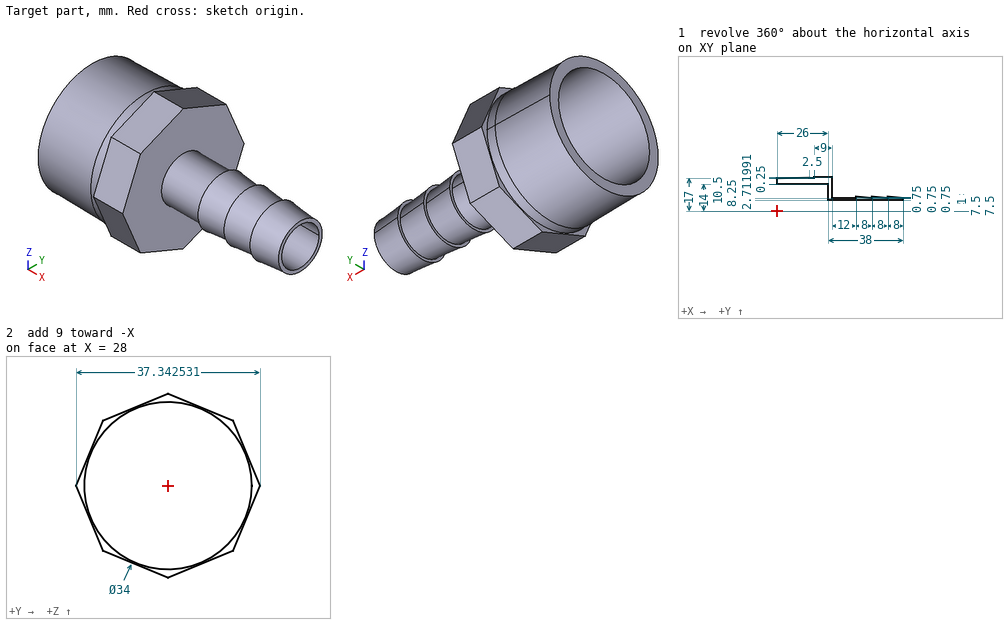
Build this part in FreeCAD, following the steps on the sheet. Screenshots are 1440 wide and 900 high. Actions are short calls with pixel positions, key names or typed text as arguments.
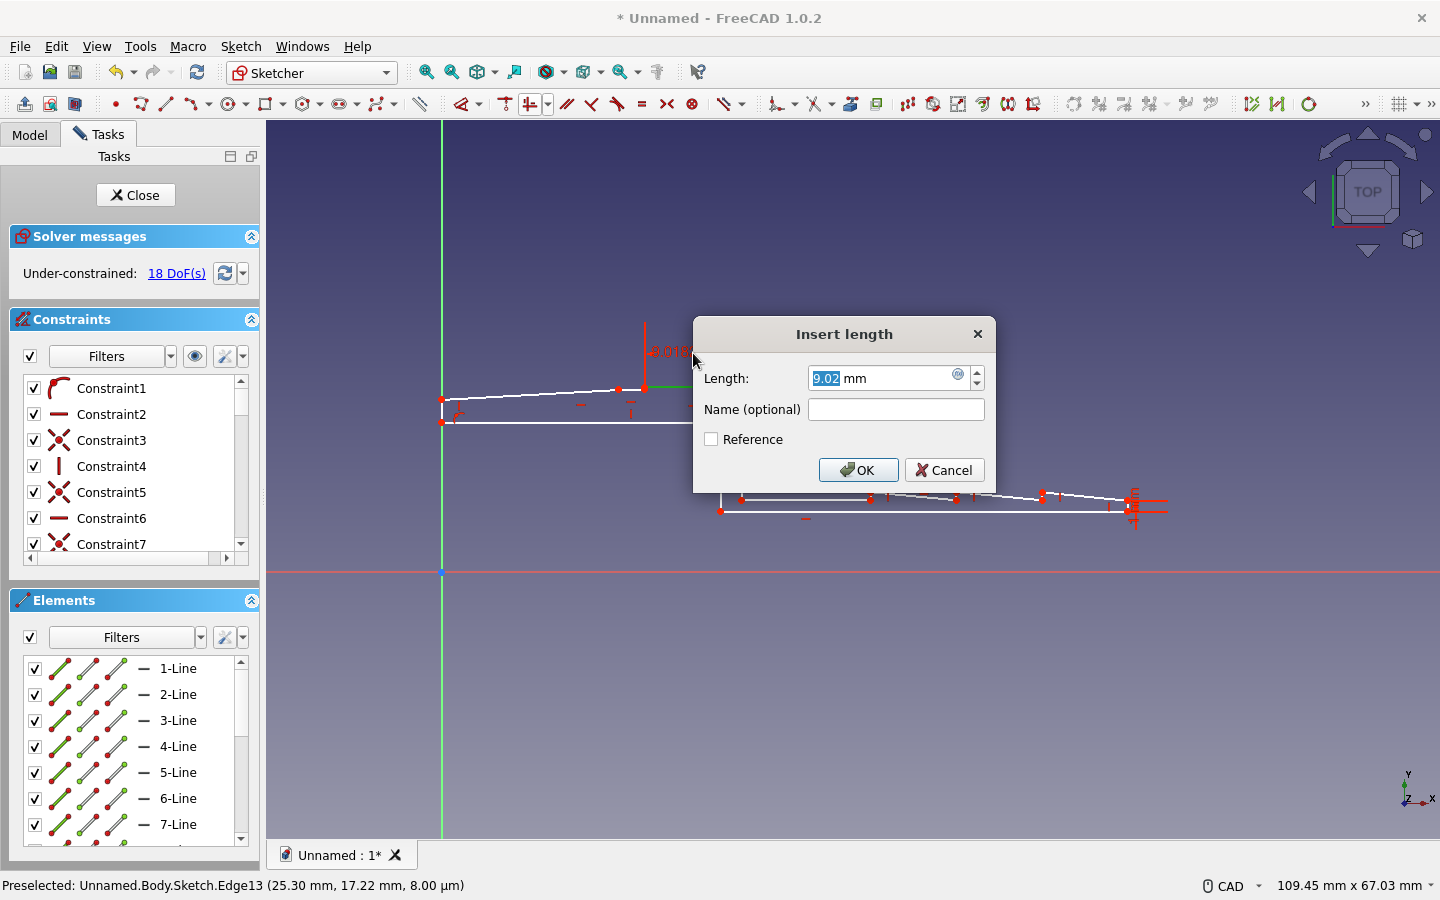
text(9)
key(Return)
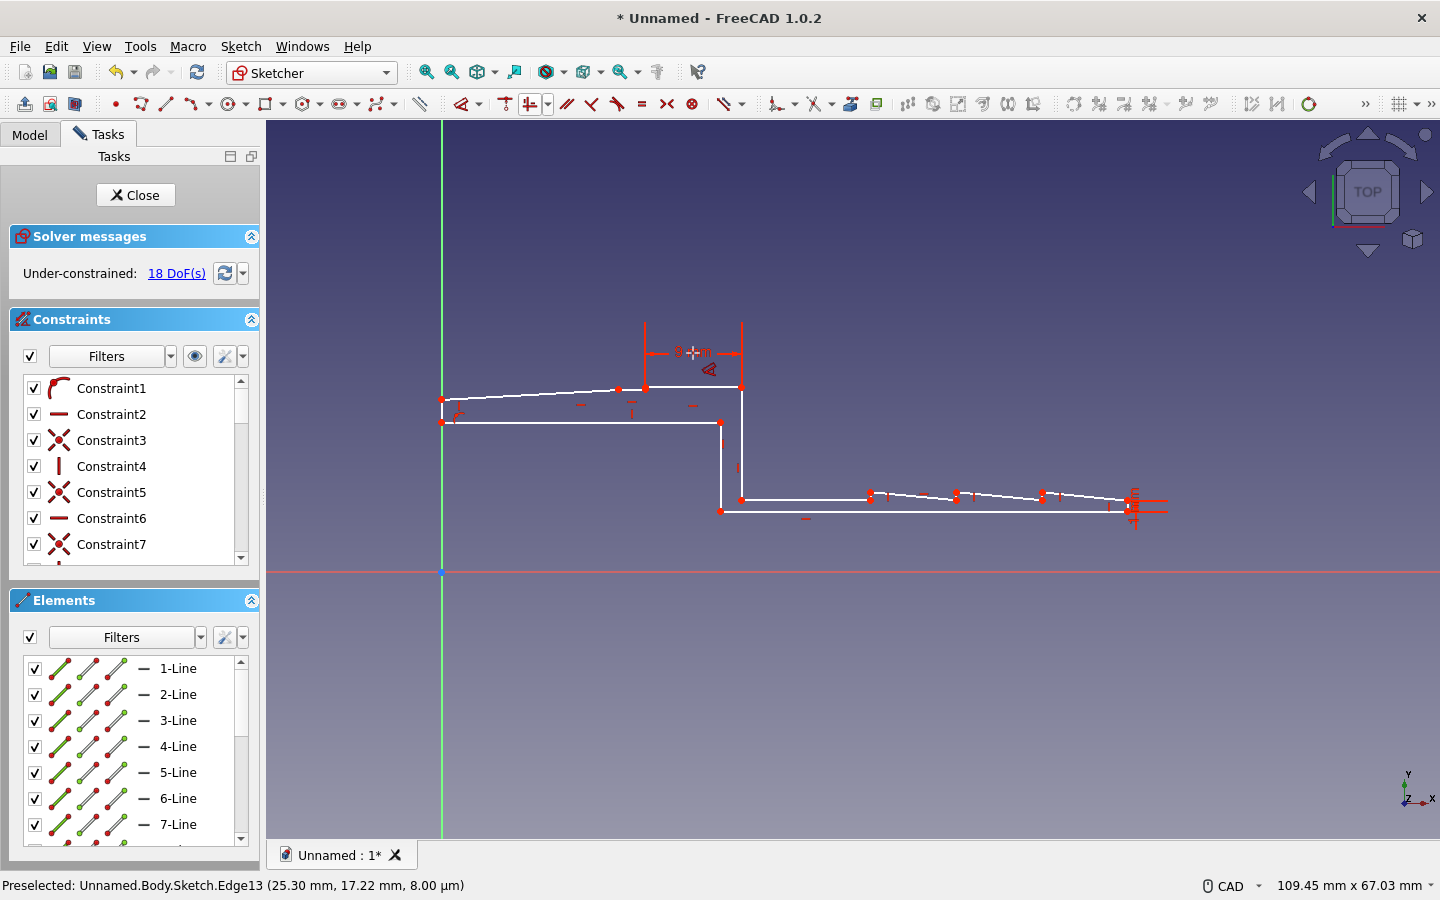
click(525, 423)
click(581, 457)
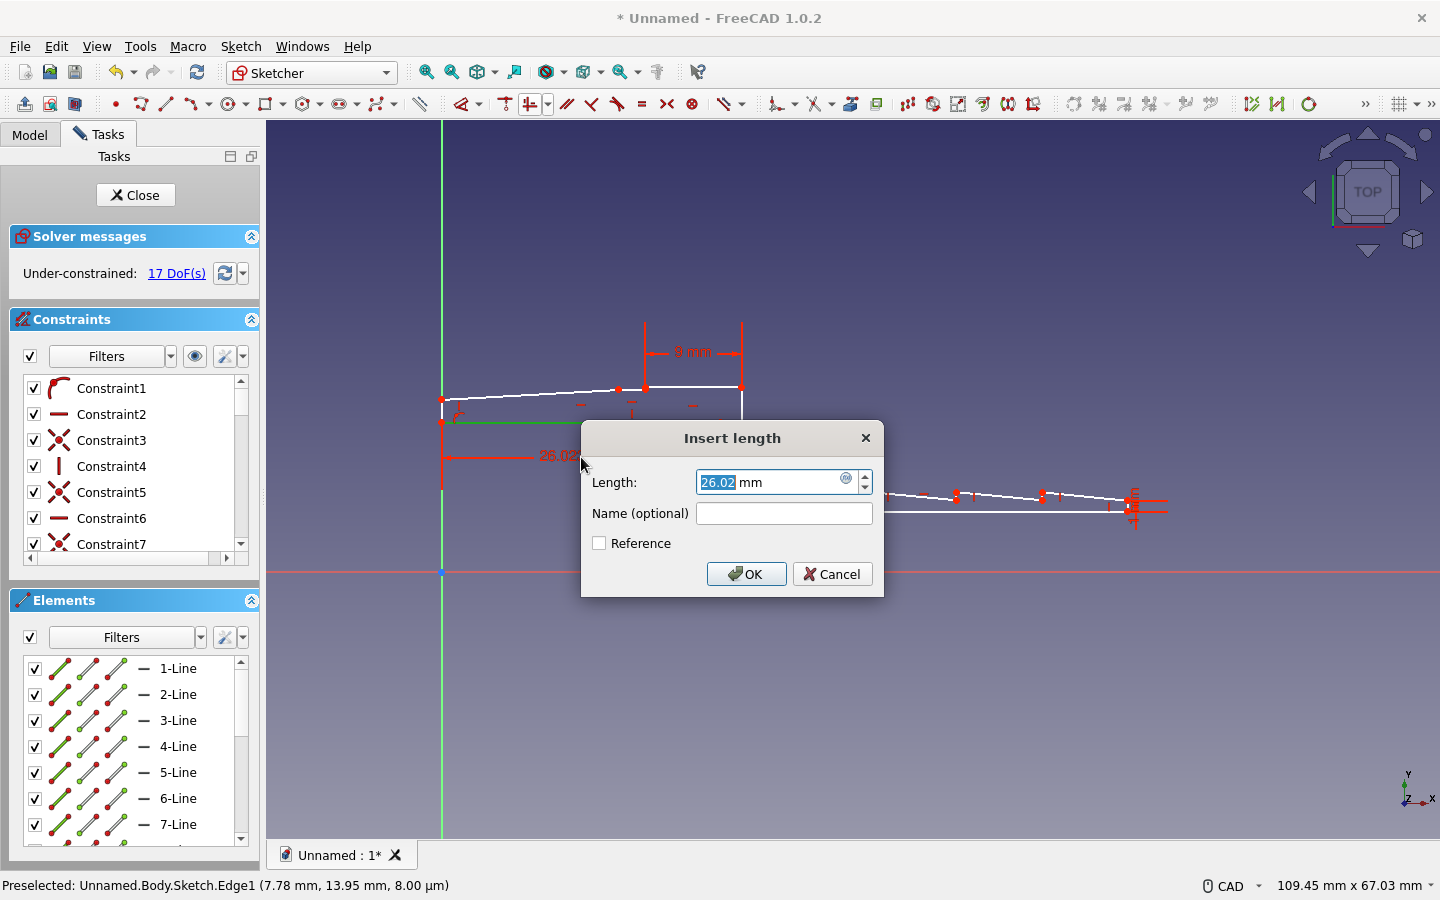
text(26)
key(Return)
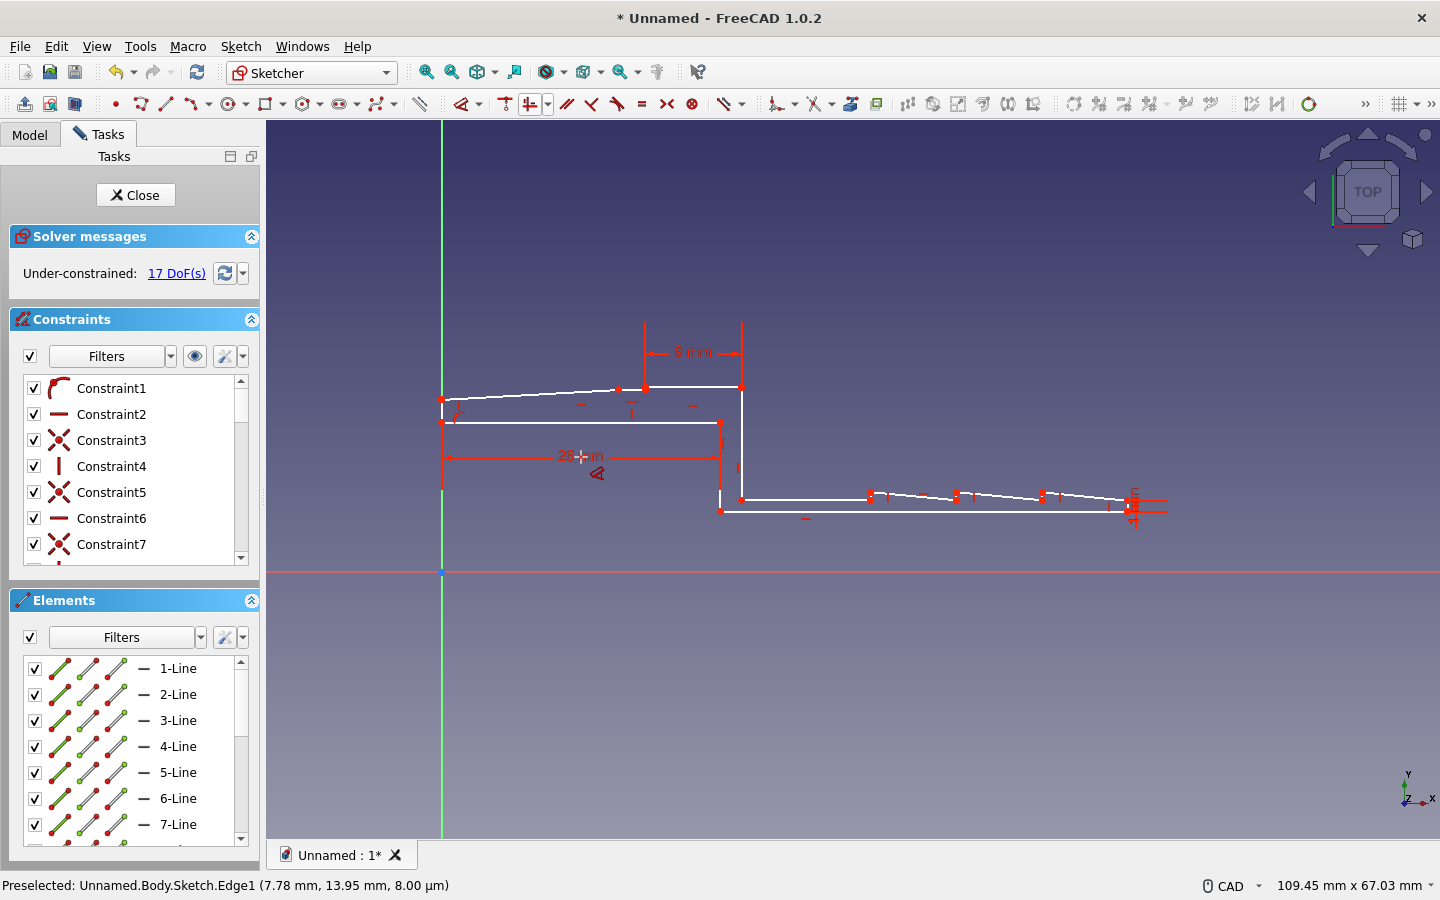
scroll(843, 512, up, 2)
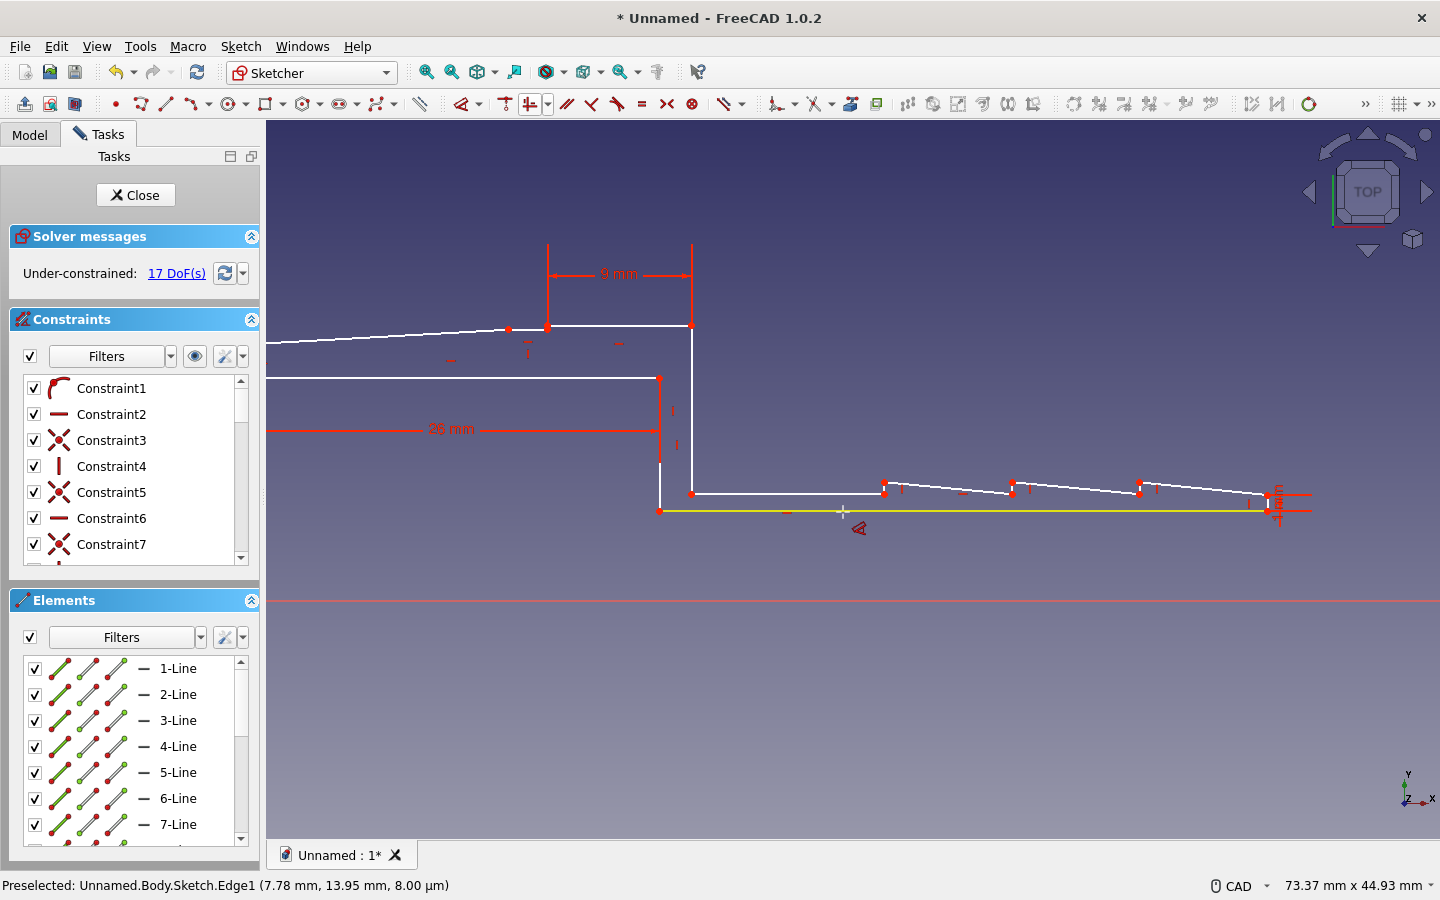
click(842, 511)
click(964, 545)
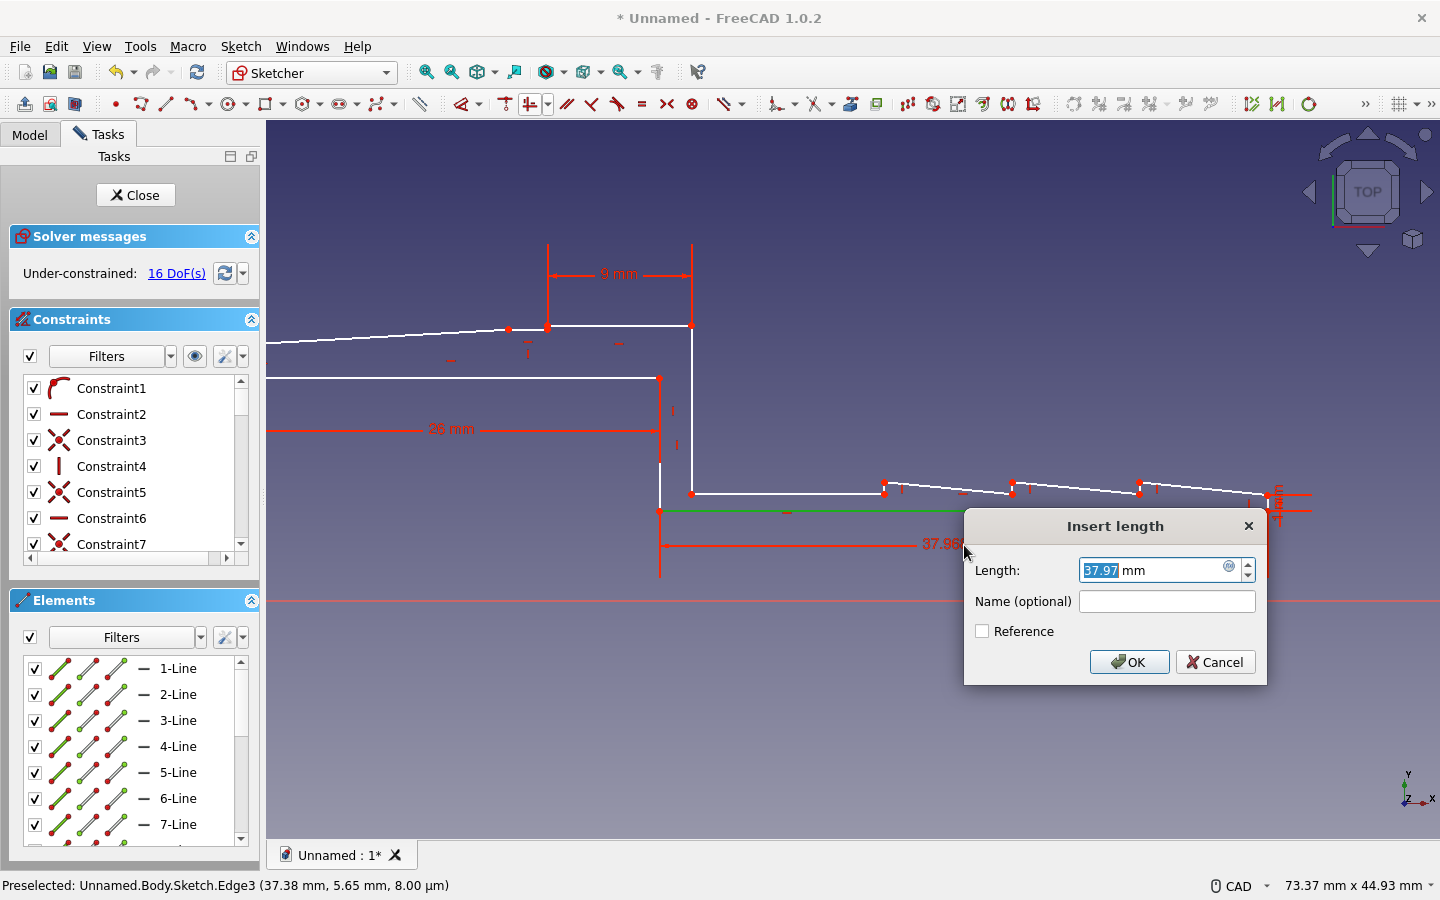
text(38)
key(Return)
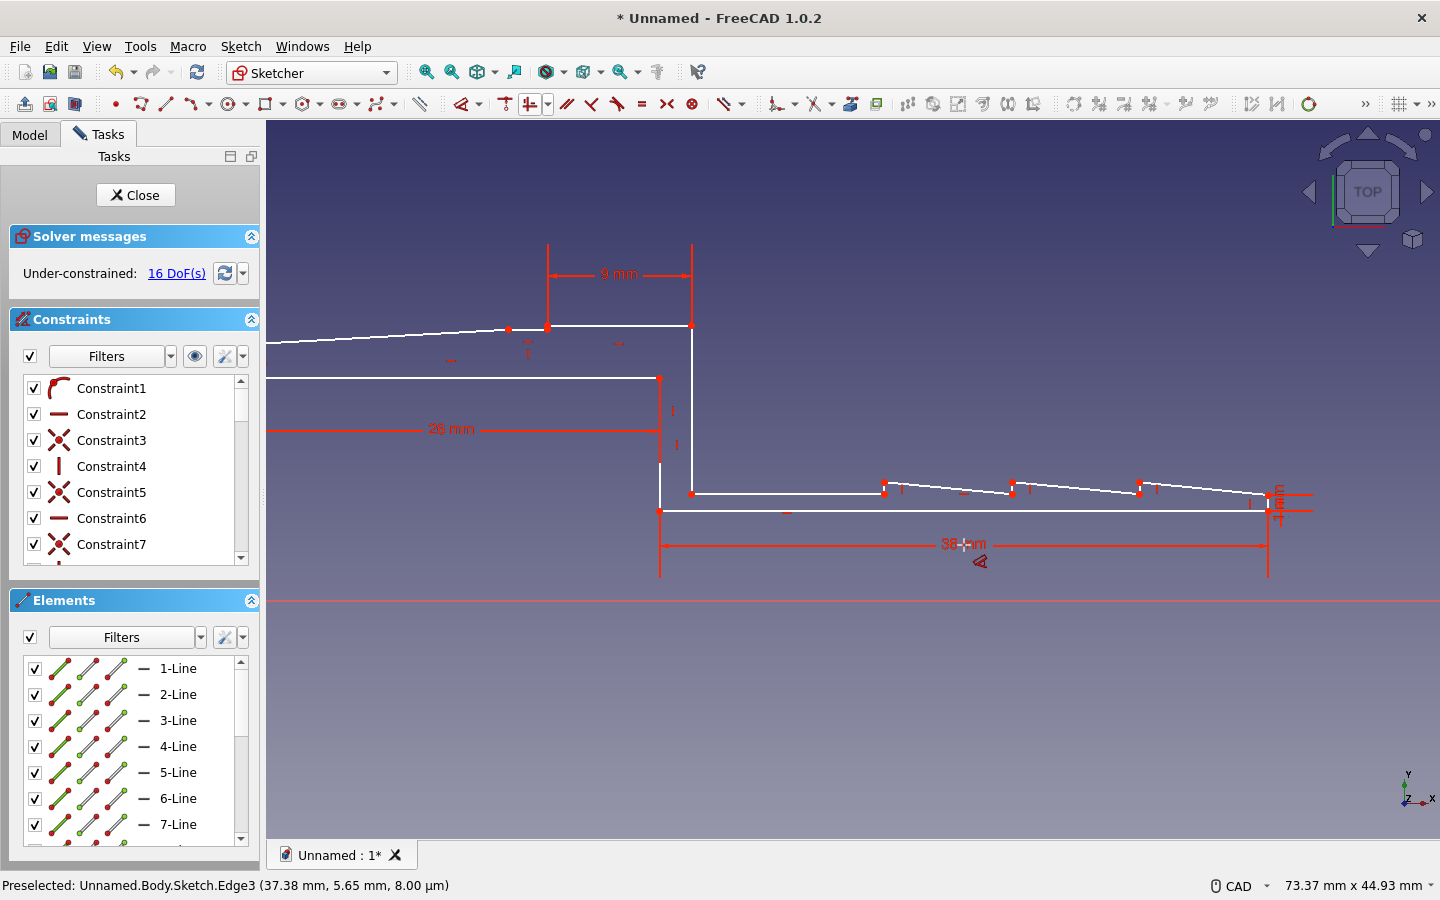
click(826, 494)
click(788, 528)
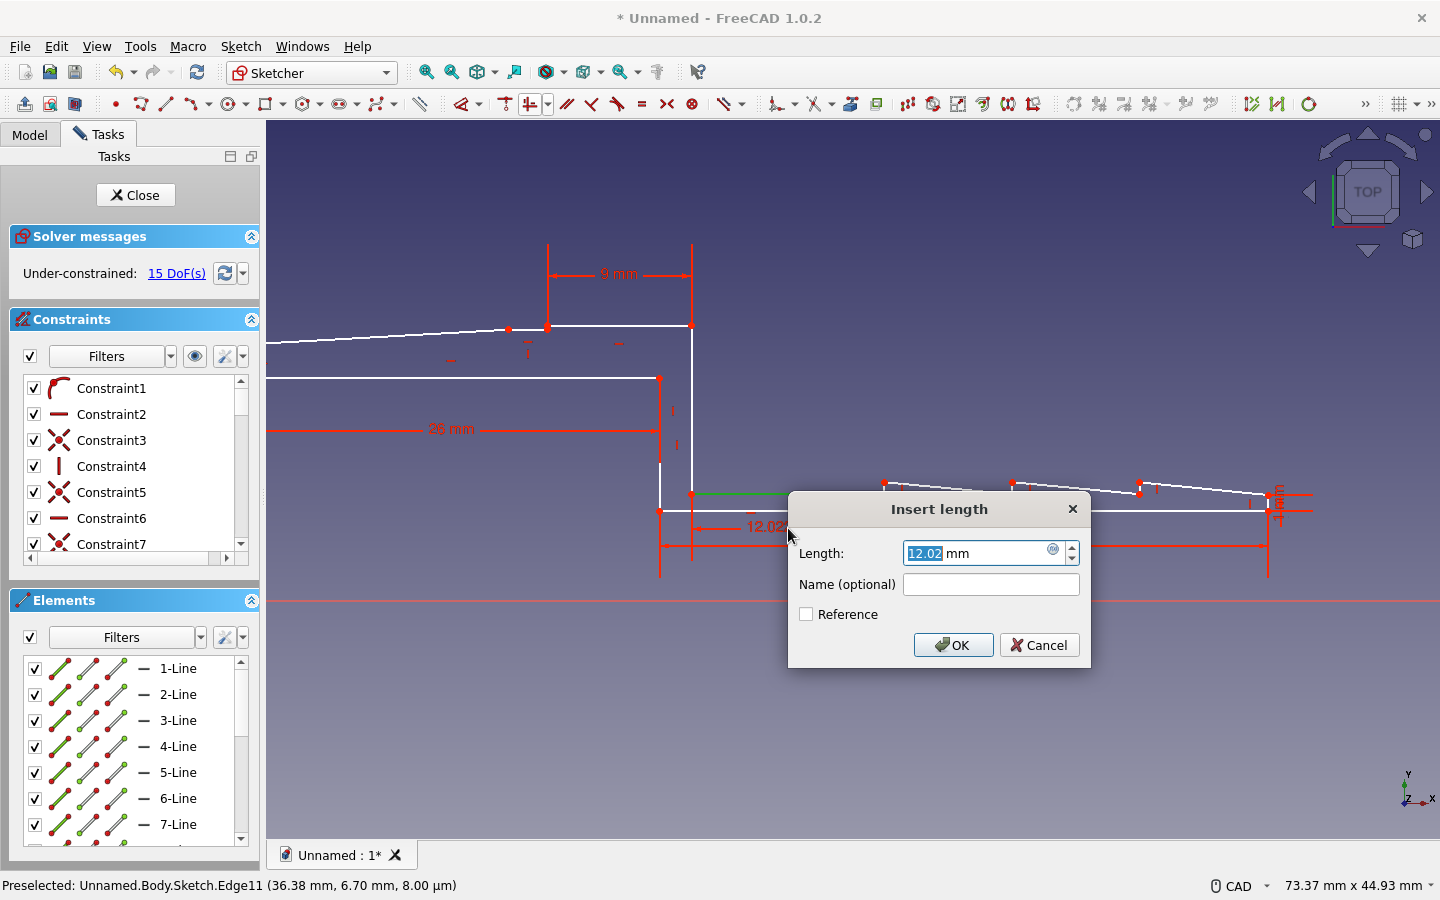
text(12)
key(Return)